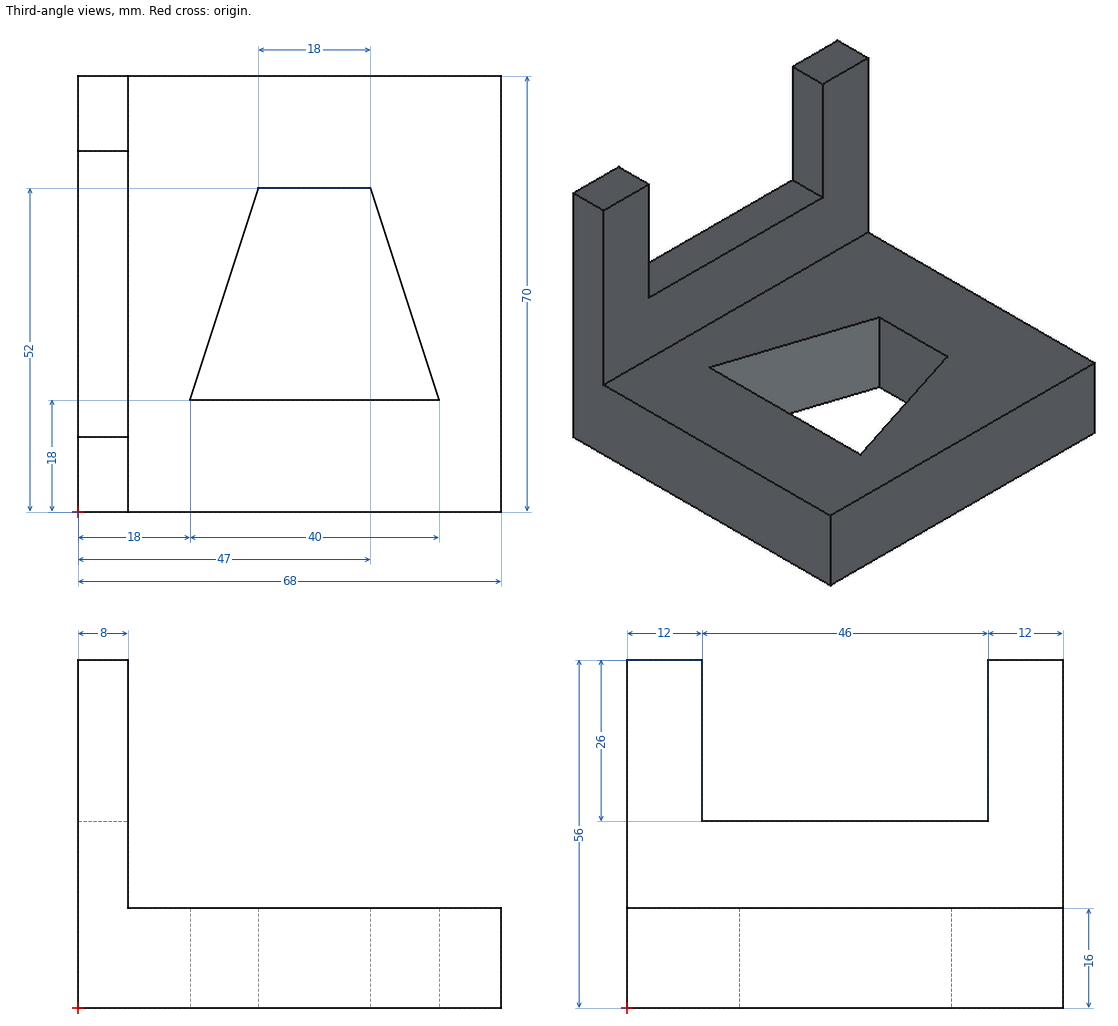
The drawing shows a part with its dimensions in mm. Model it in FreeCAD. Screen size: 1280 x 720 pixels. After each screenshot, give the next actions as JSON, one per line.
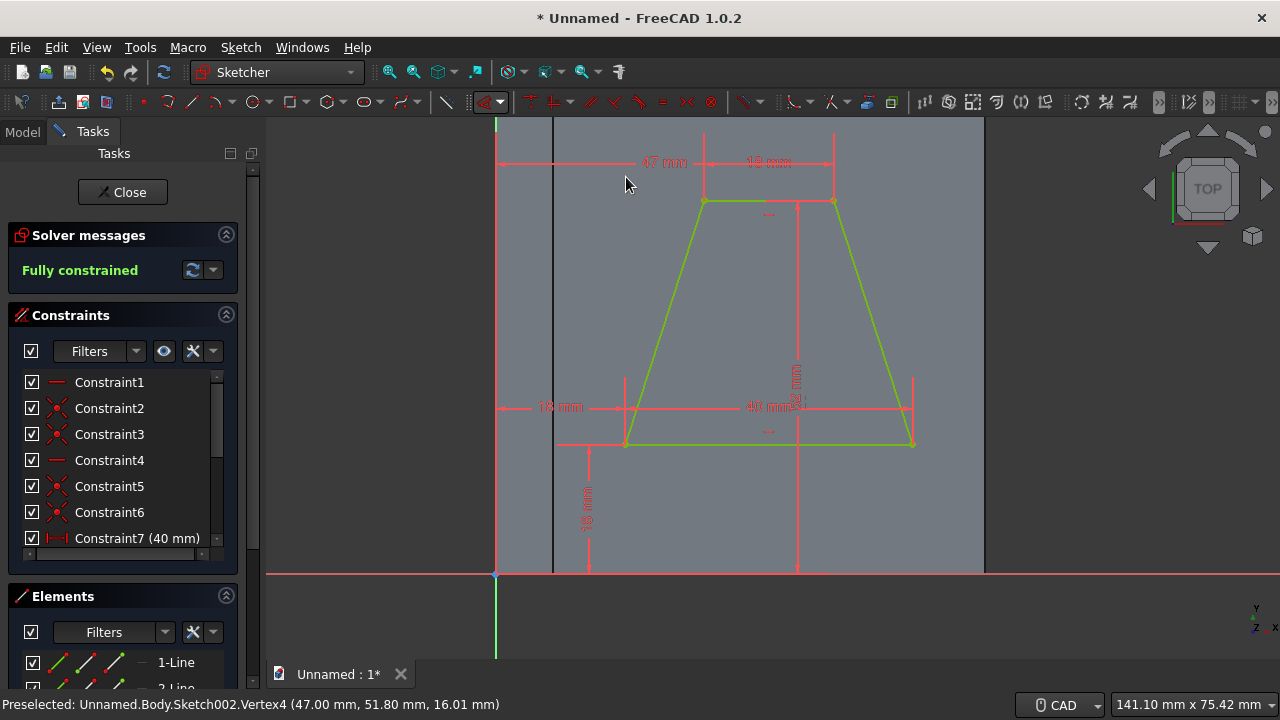
{"action": "left_click", "coordinate": [123, 192]}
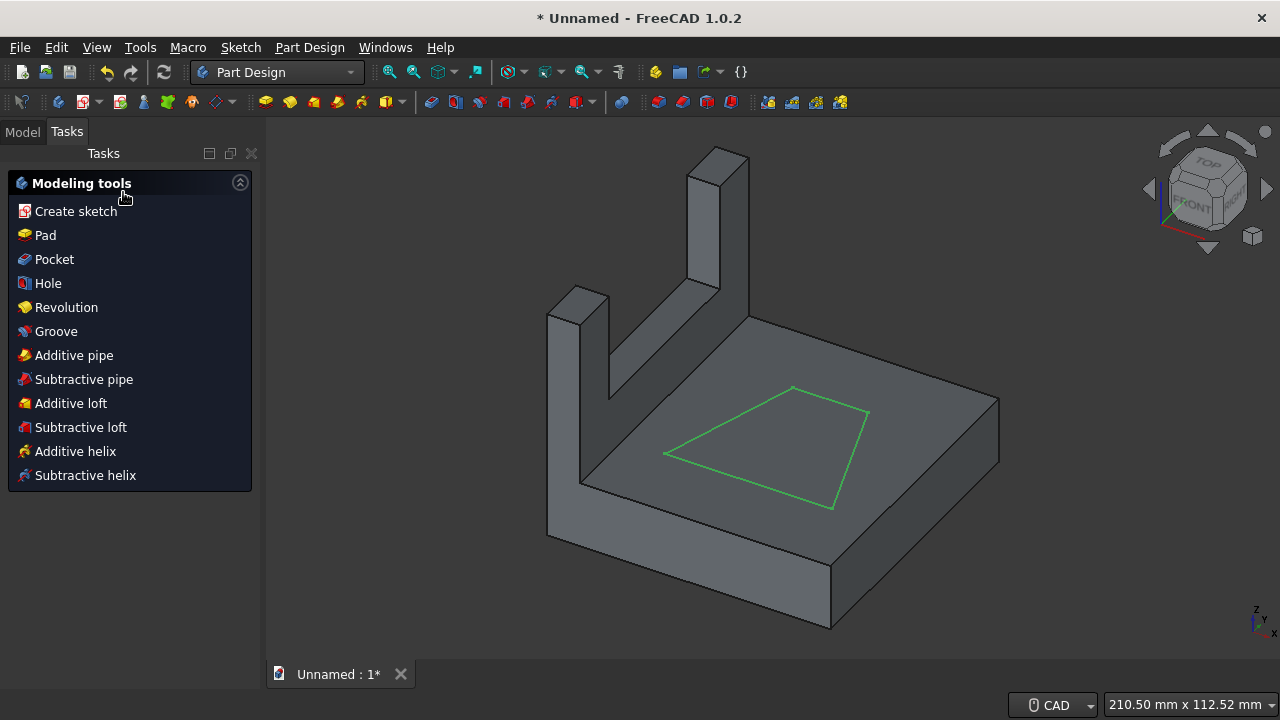
{"action": "left_click", "coordinate": [432, 102]}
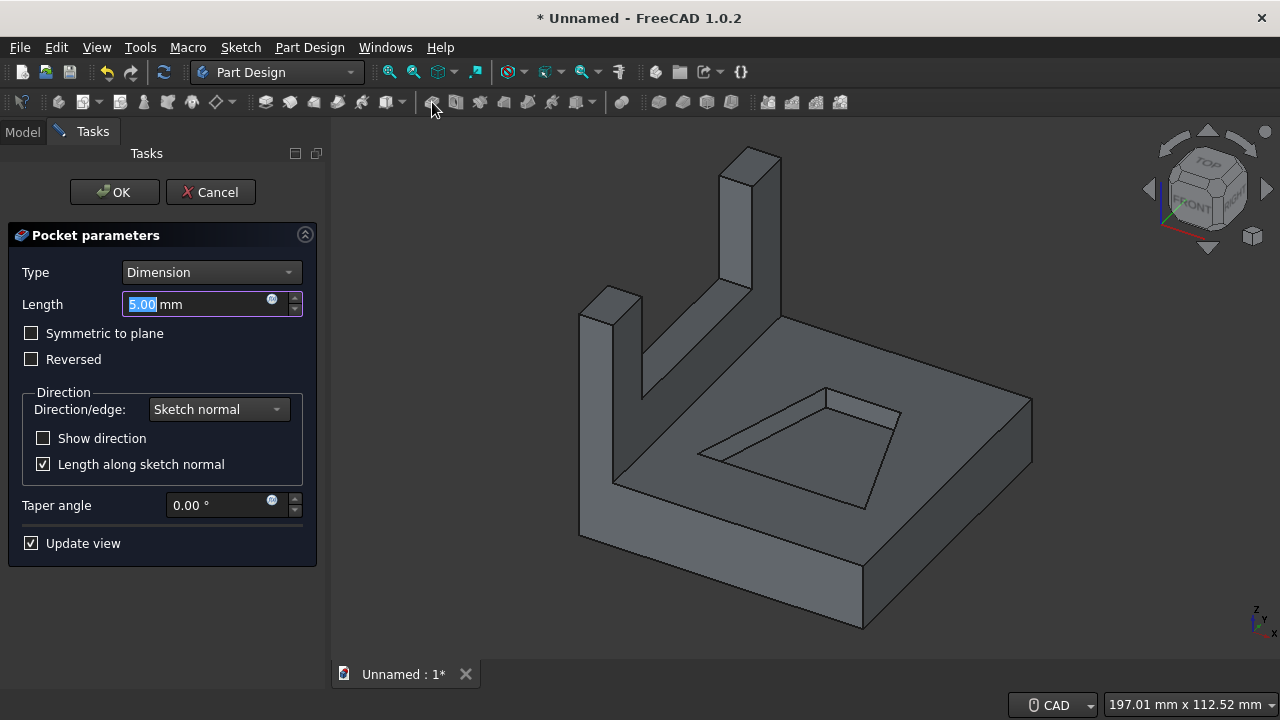
{"action": "type", "text": "18"}
{"action": "key", "text": "Tab"}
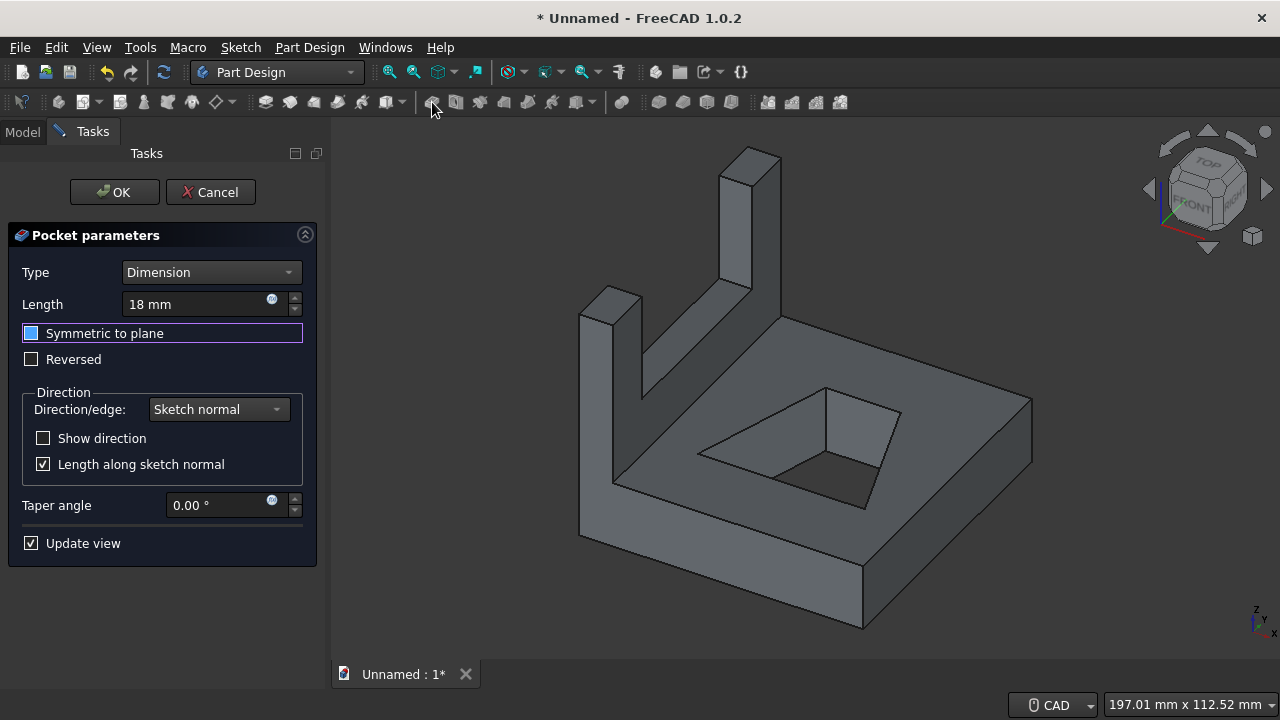
{"action": "left_click", "coordinate": [115, 192]}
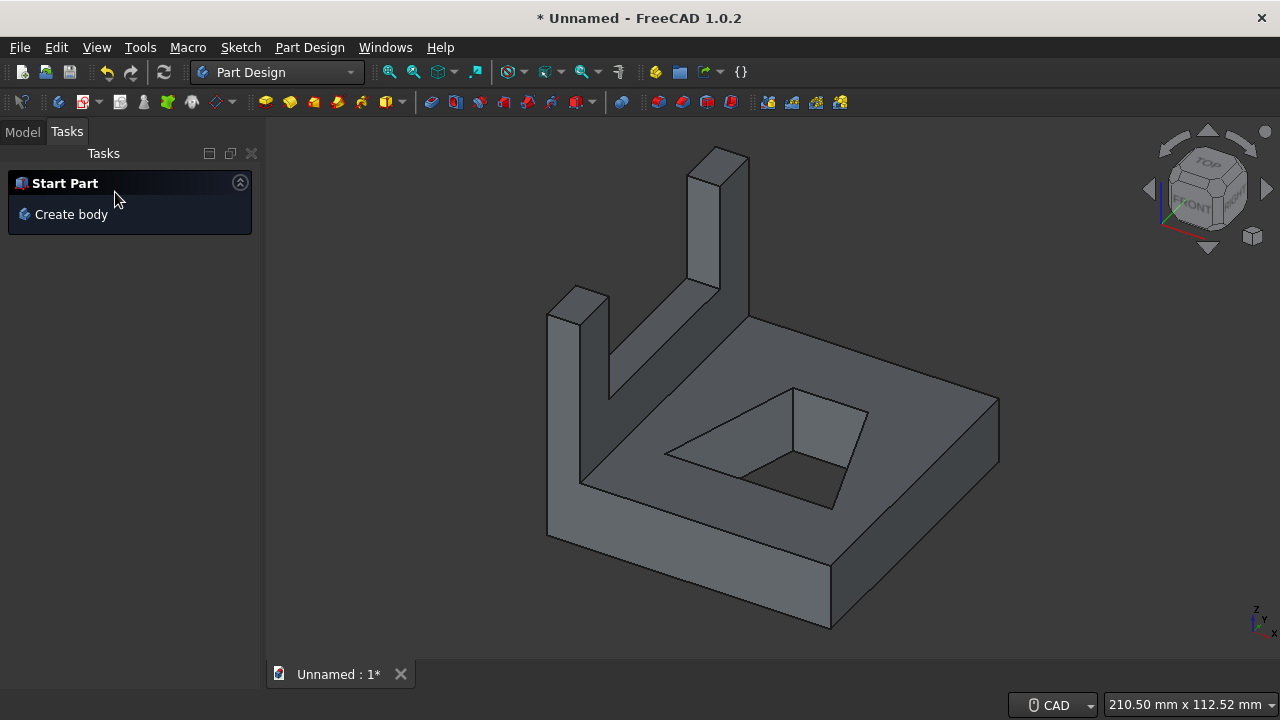
{"action": "key", "text": "0"}